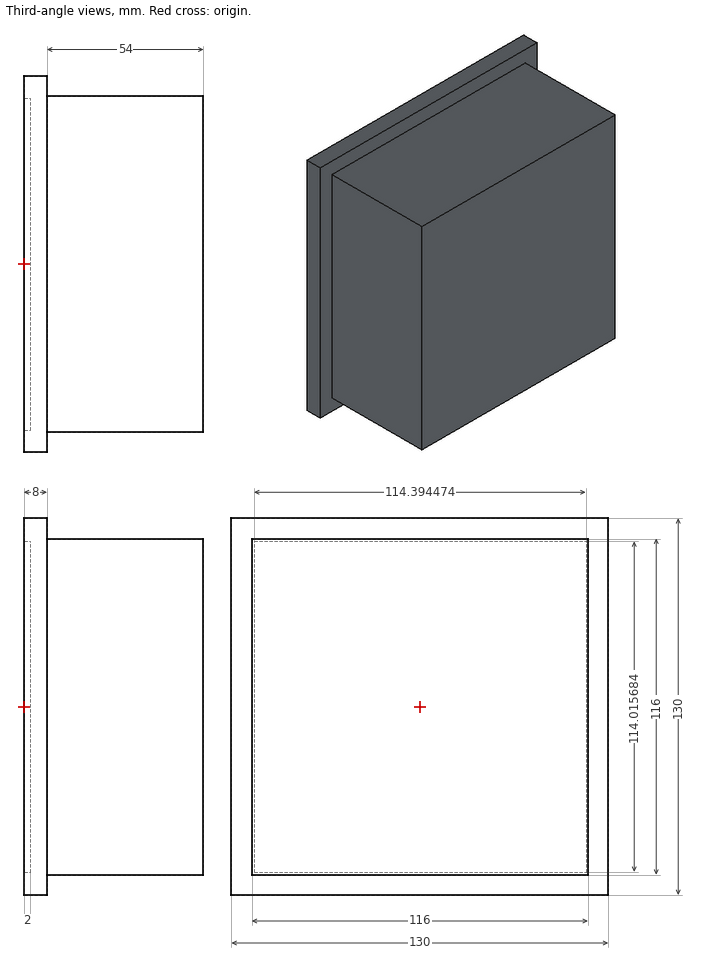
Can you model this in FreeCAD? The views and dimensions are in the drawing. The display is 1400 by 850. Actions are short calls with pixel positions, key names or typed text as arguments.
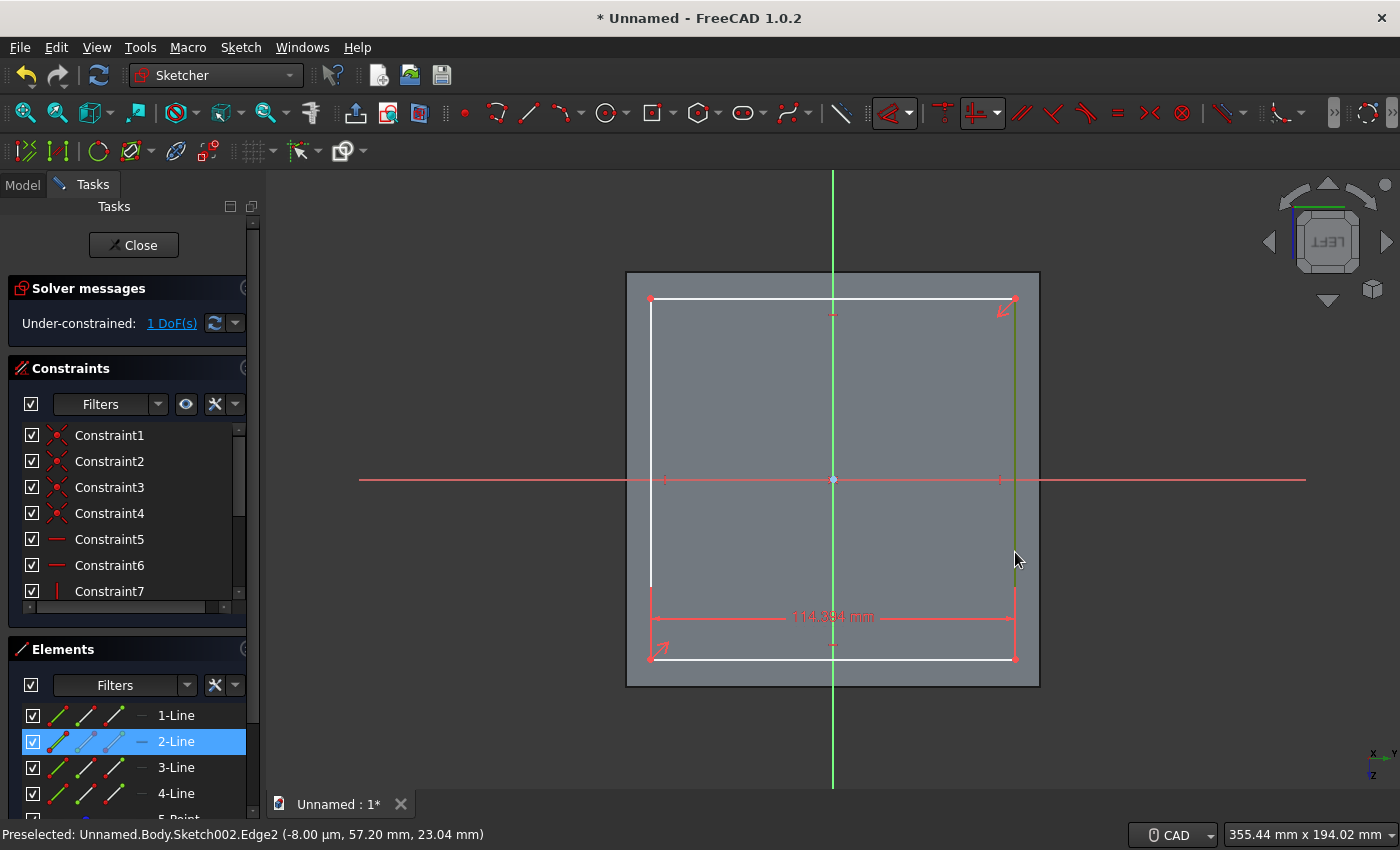
click(912, 114)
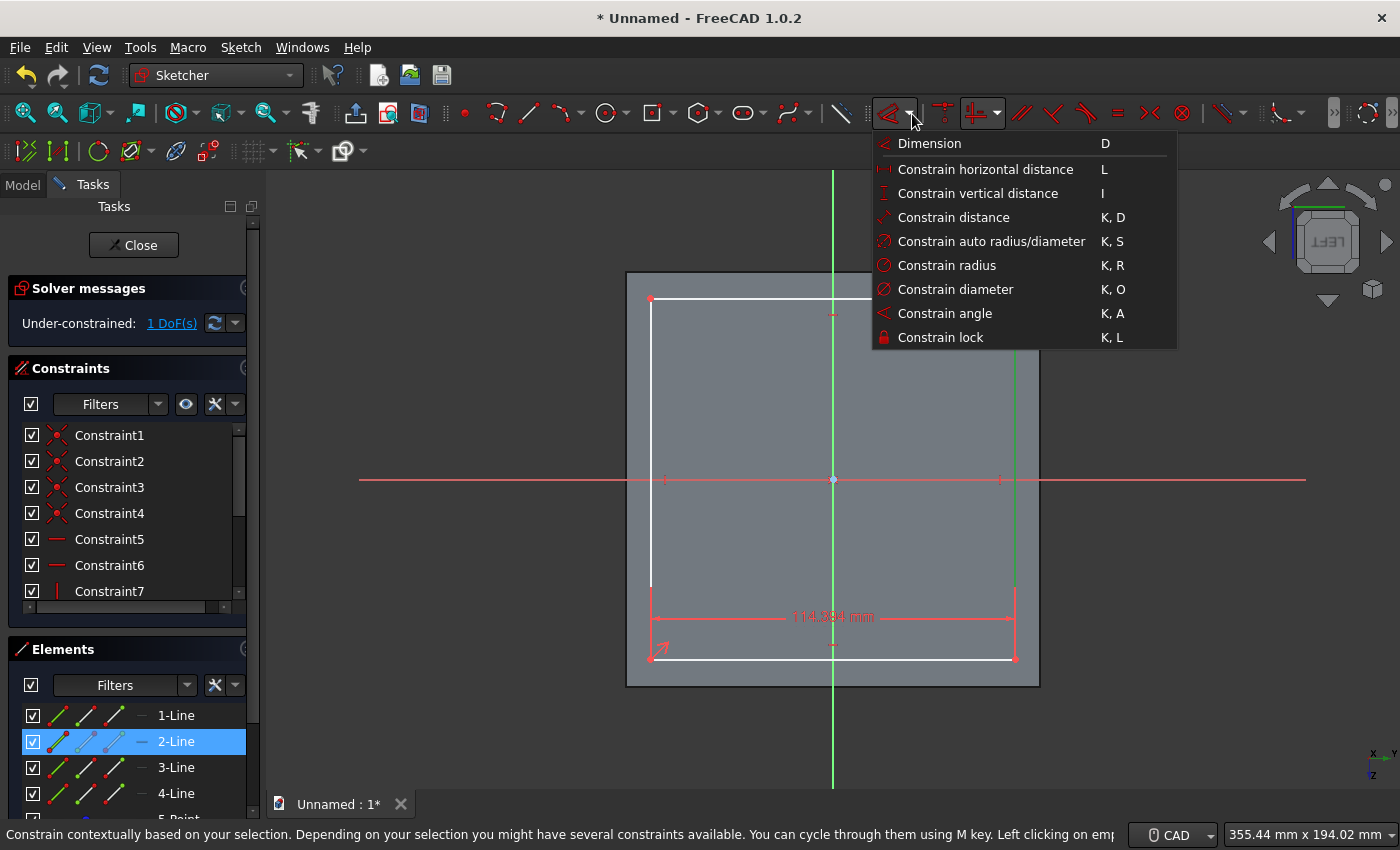
click(1025, 193)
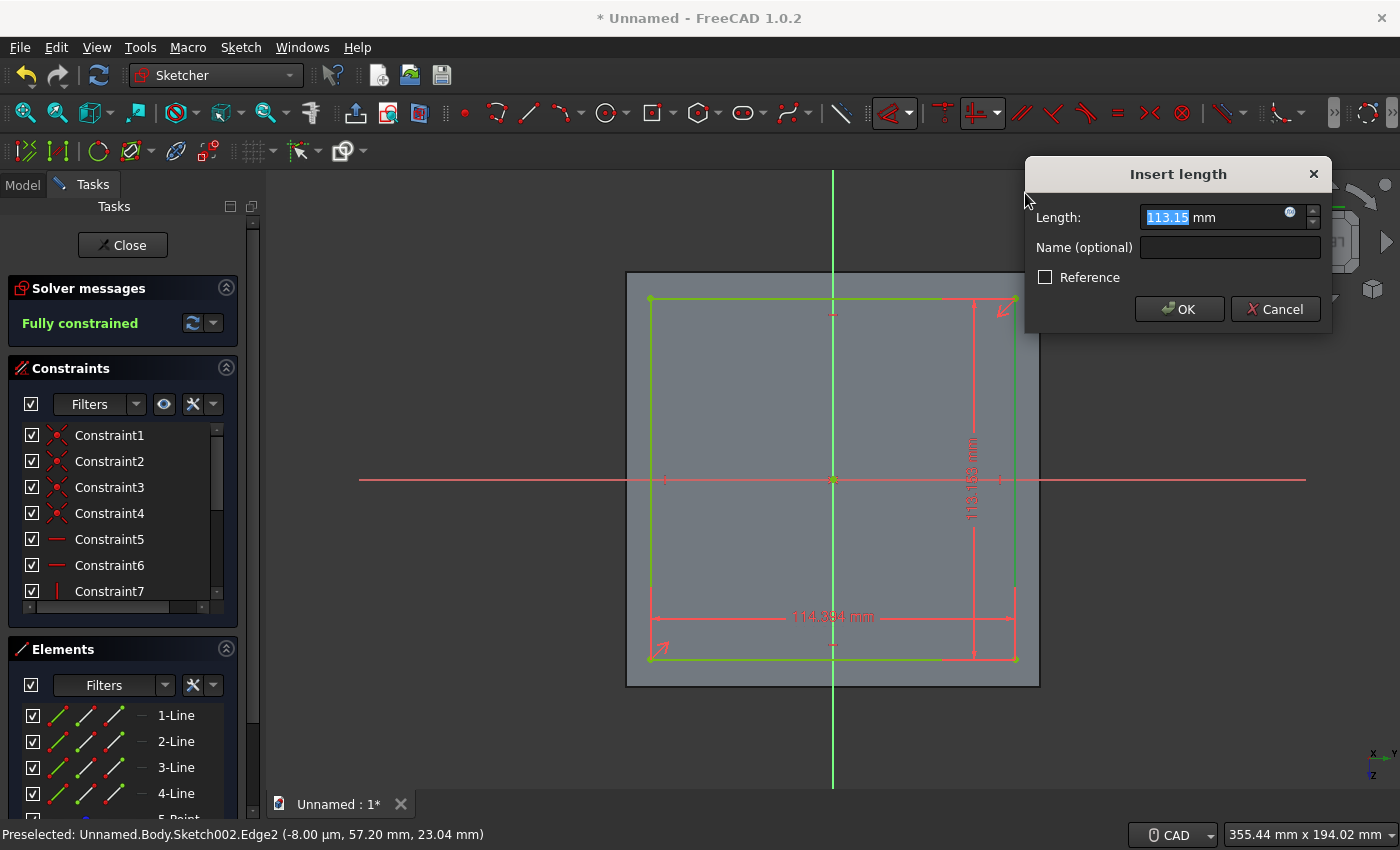
text(114.015684)
key(Return)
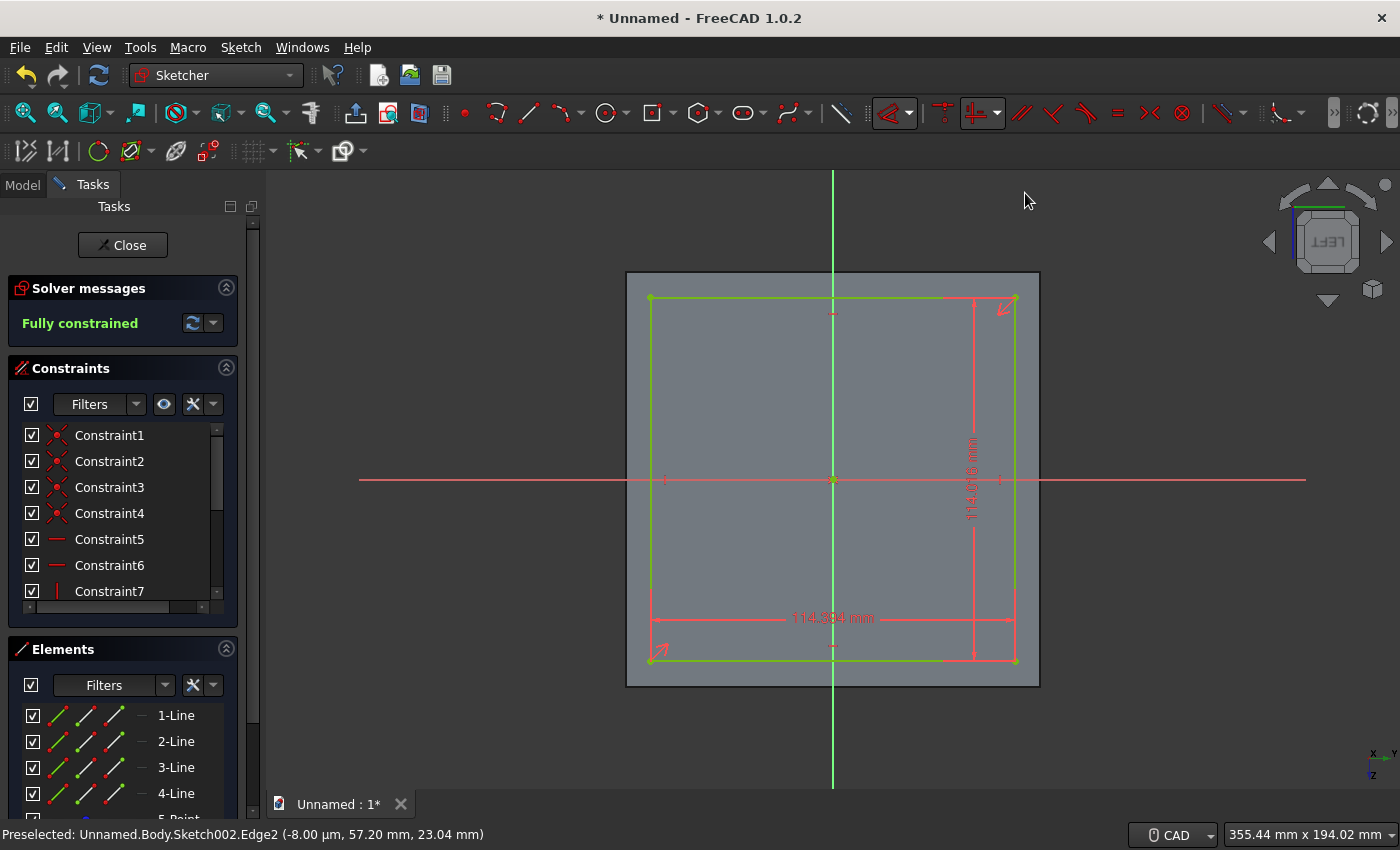
click(123, 245)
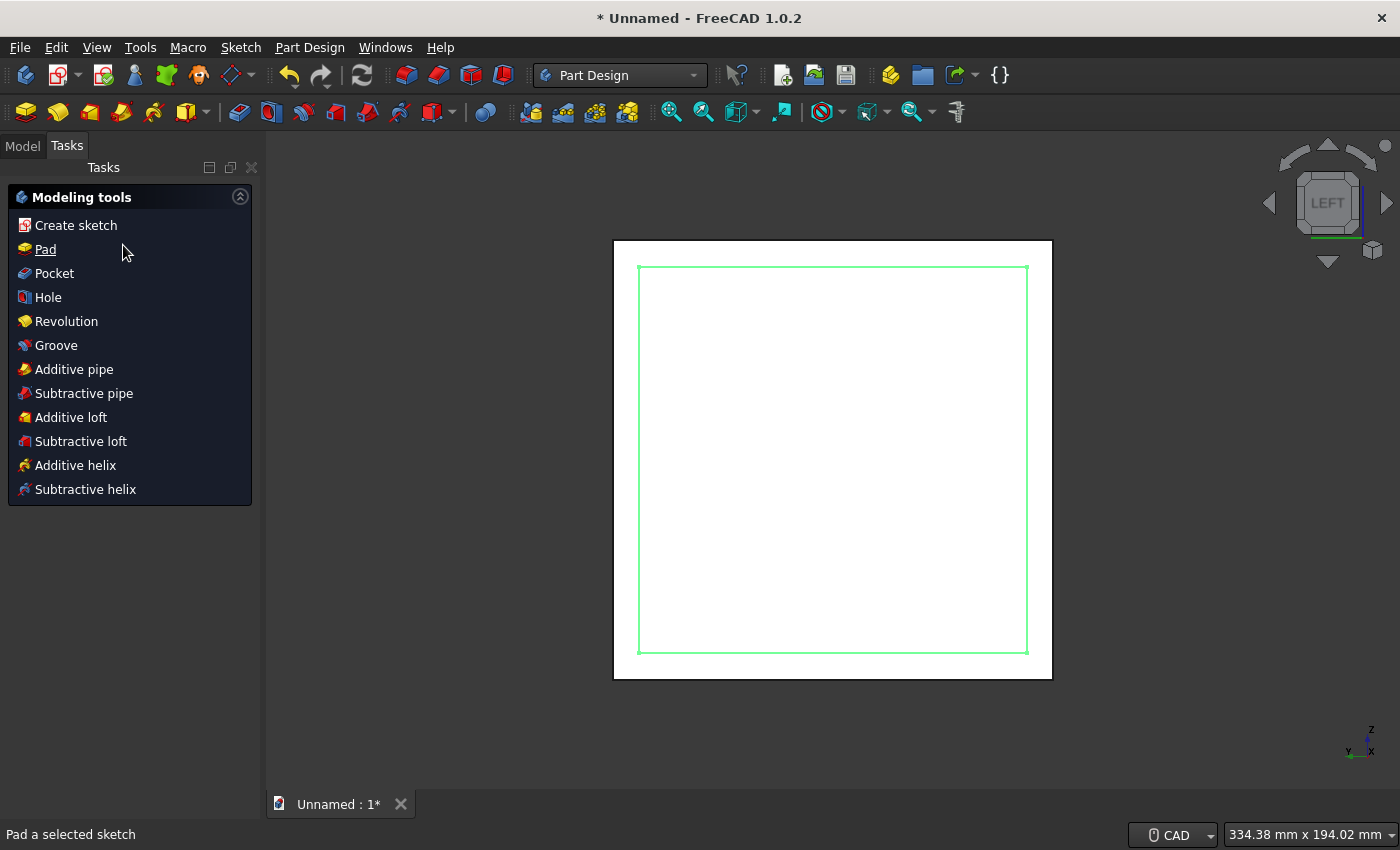
click(240, 112)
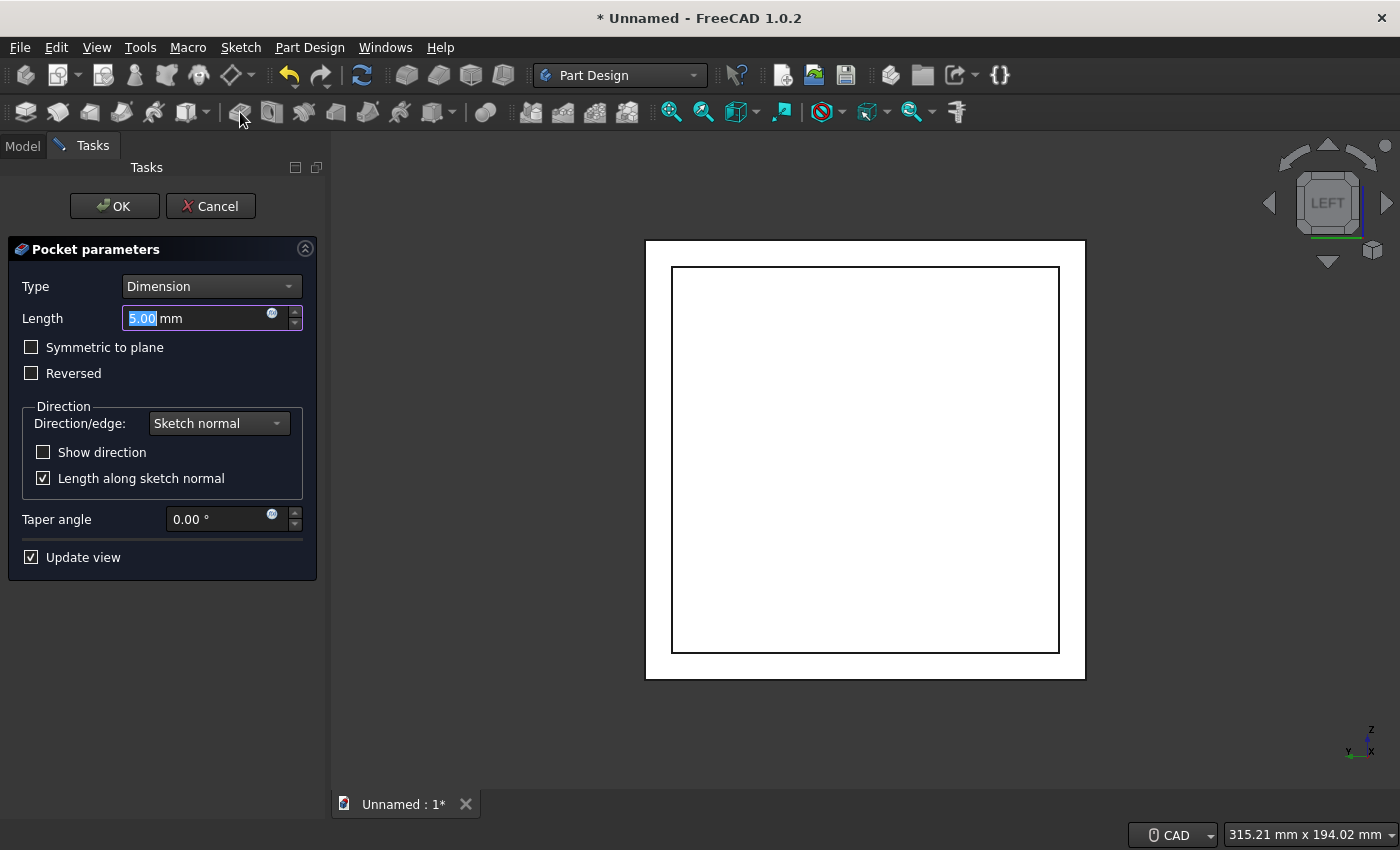
text(2)
key(Tab)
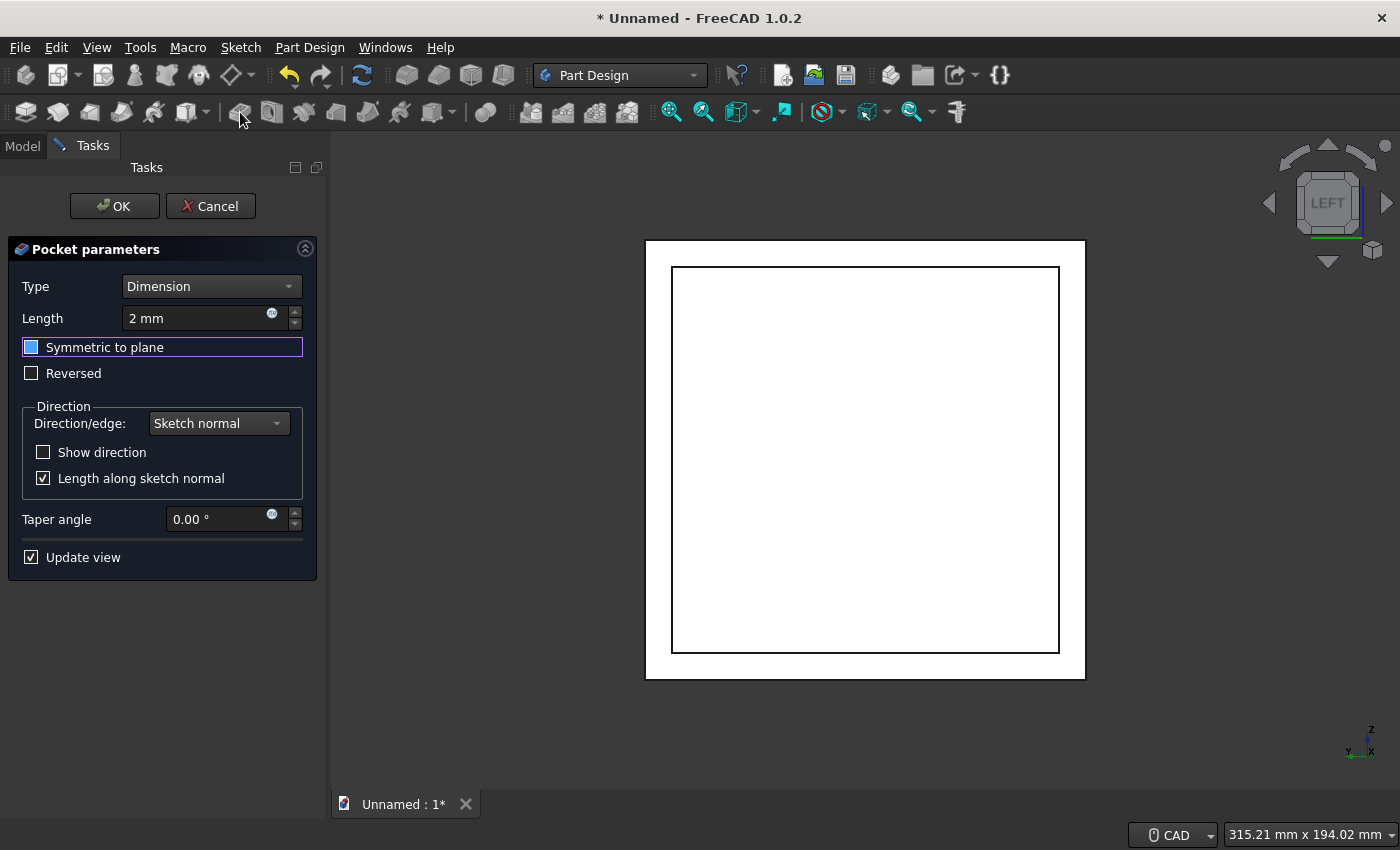
click(115, 206)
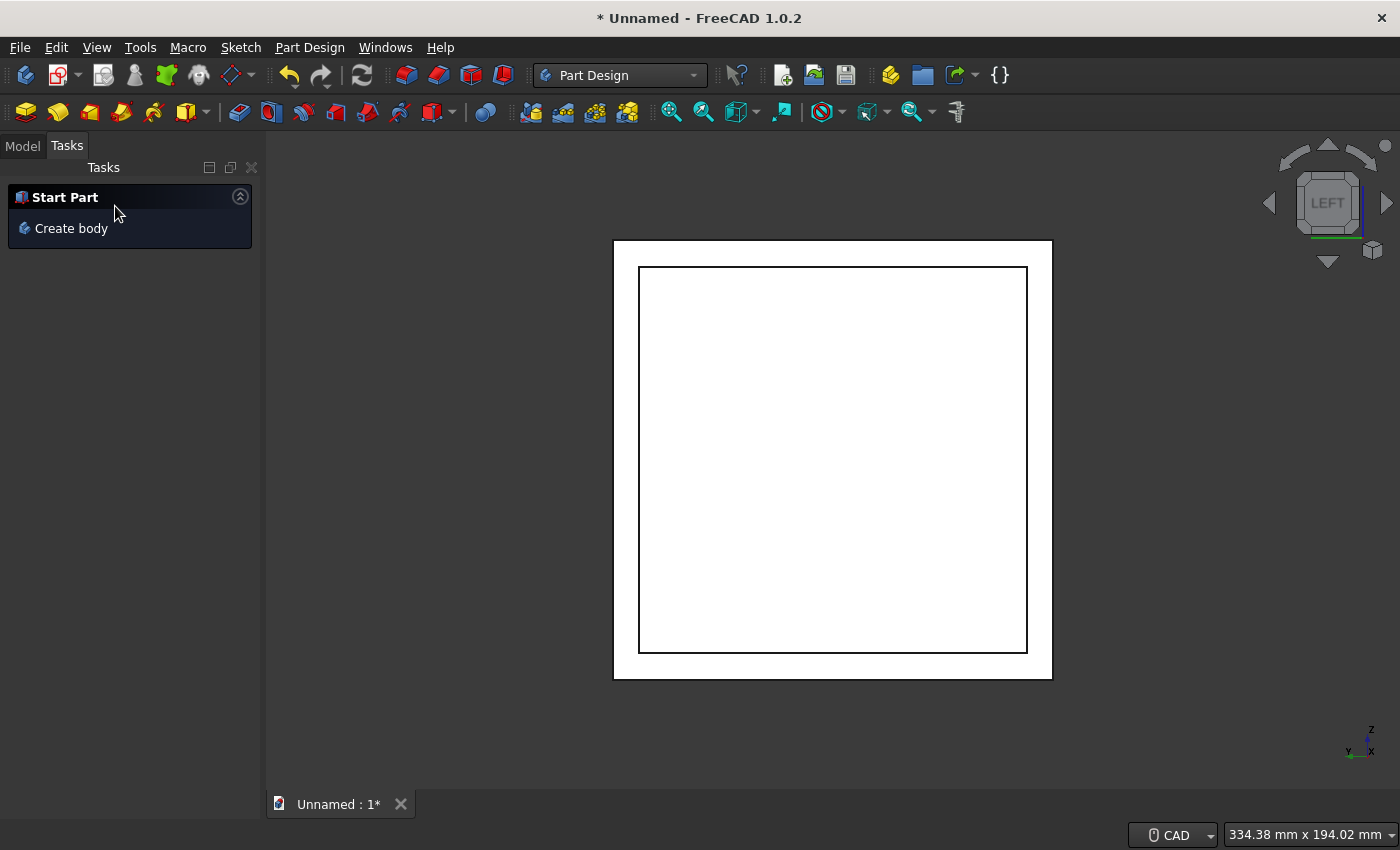
key(0)